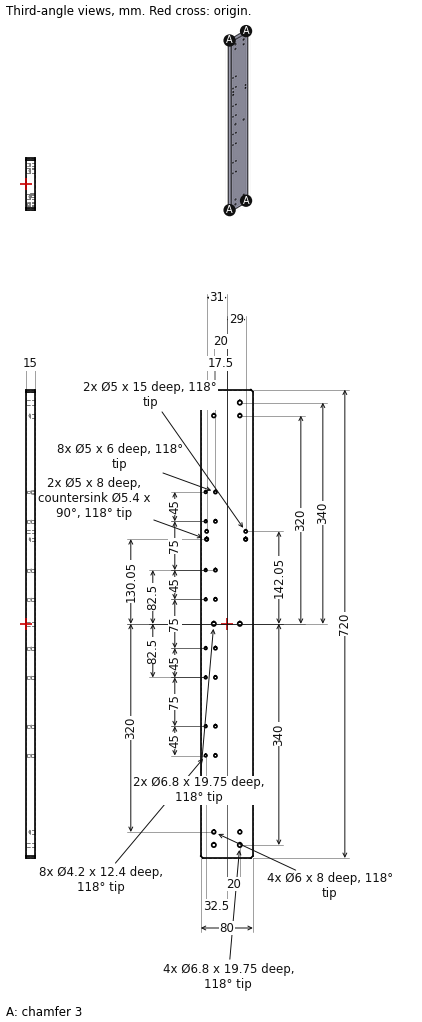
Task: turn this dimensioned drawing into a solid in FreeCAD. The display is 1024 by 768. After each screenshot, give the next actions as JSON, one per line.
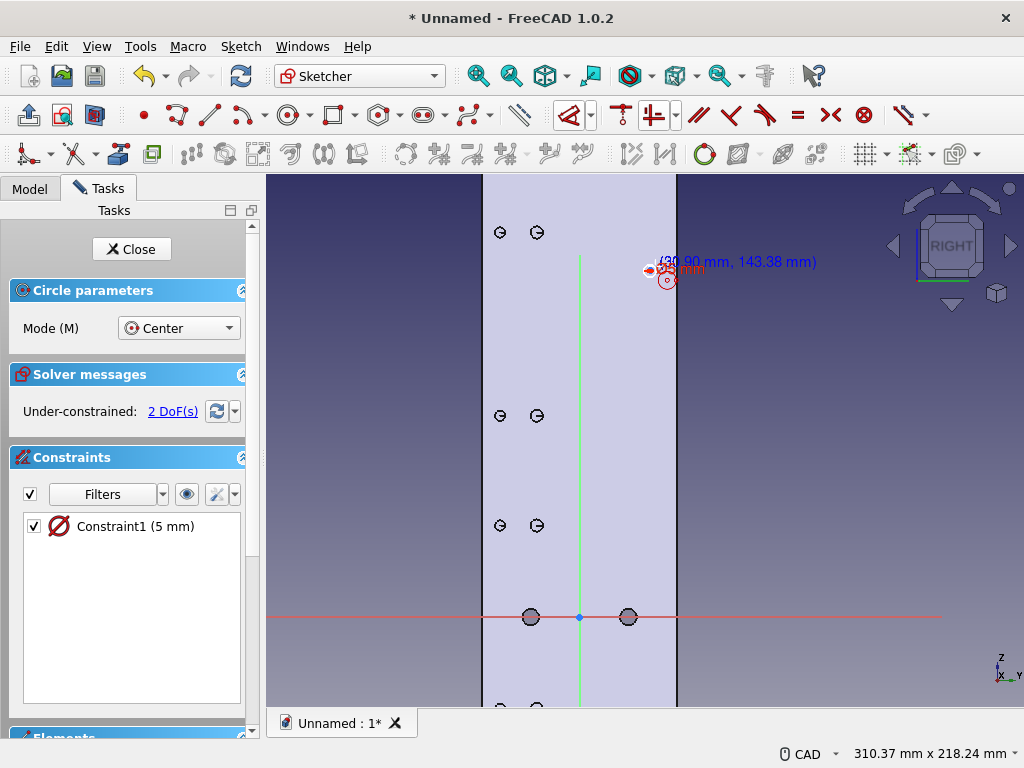
{"action": "scroll", "coordinate": [504, 270], "scroll_direction": "up", "scroll_amount": 7}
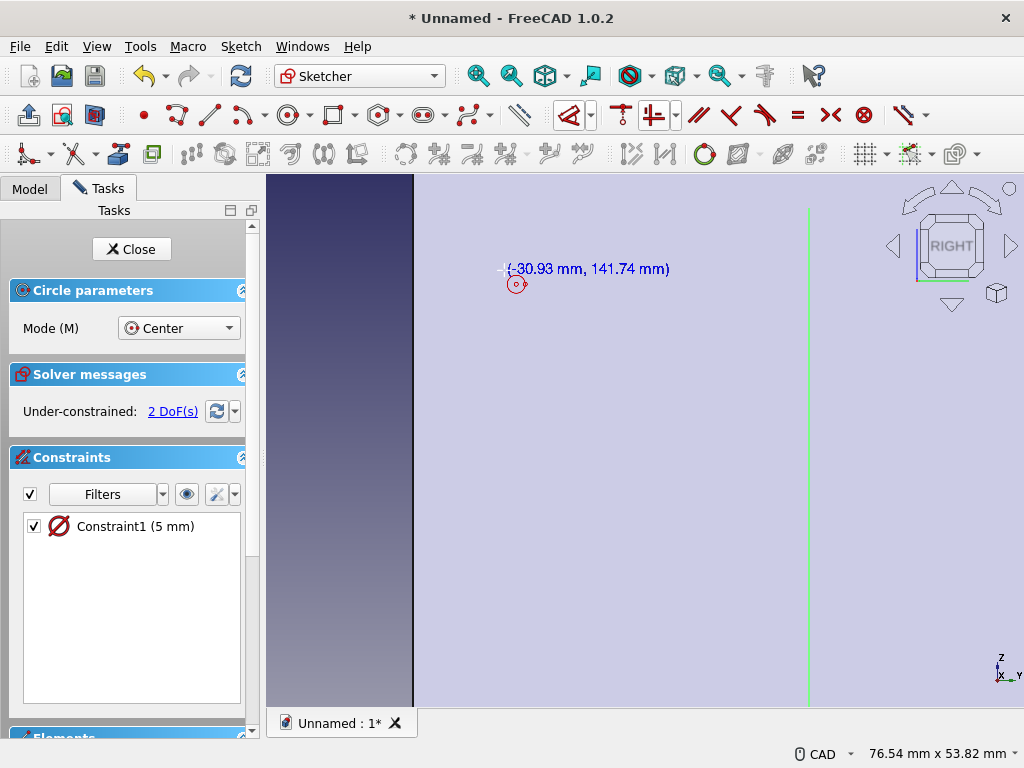
{"action": "scroll", "coordinate": [504, 270], "scroll_direction": "down", "scroll_amount": 7}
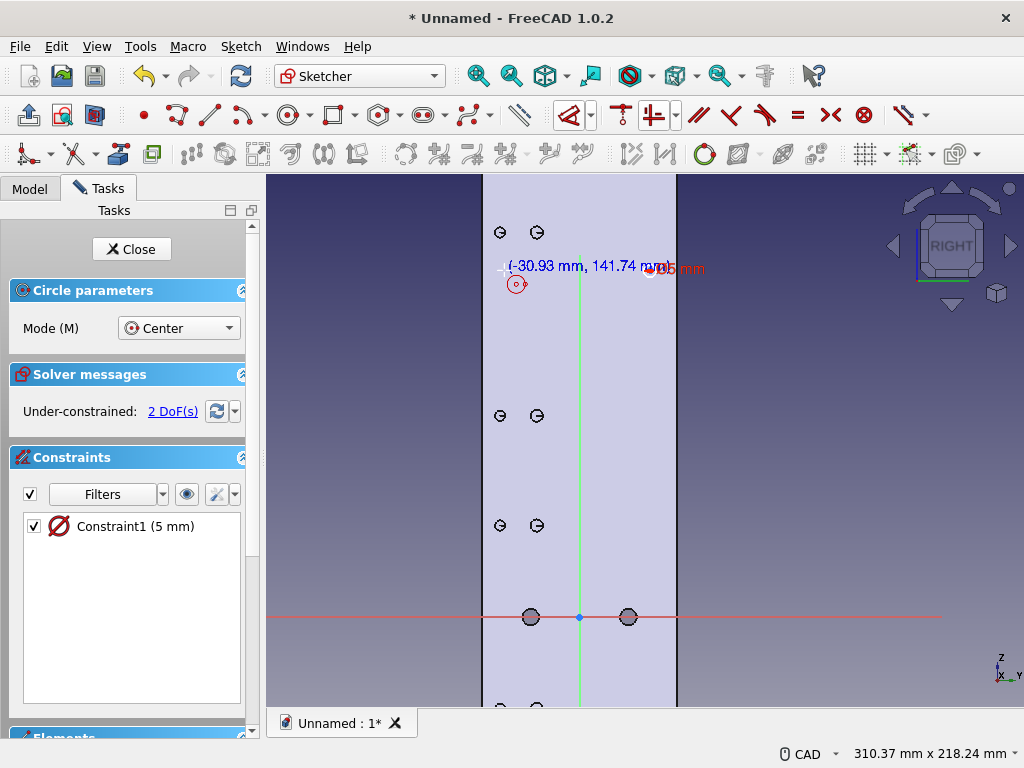
{"action": "left_click", "coordinate": [504, 270]}
{"action": "mouse_move", "coordinate": [508, 266]}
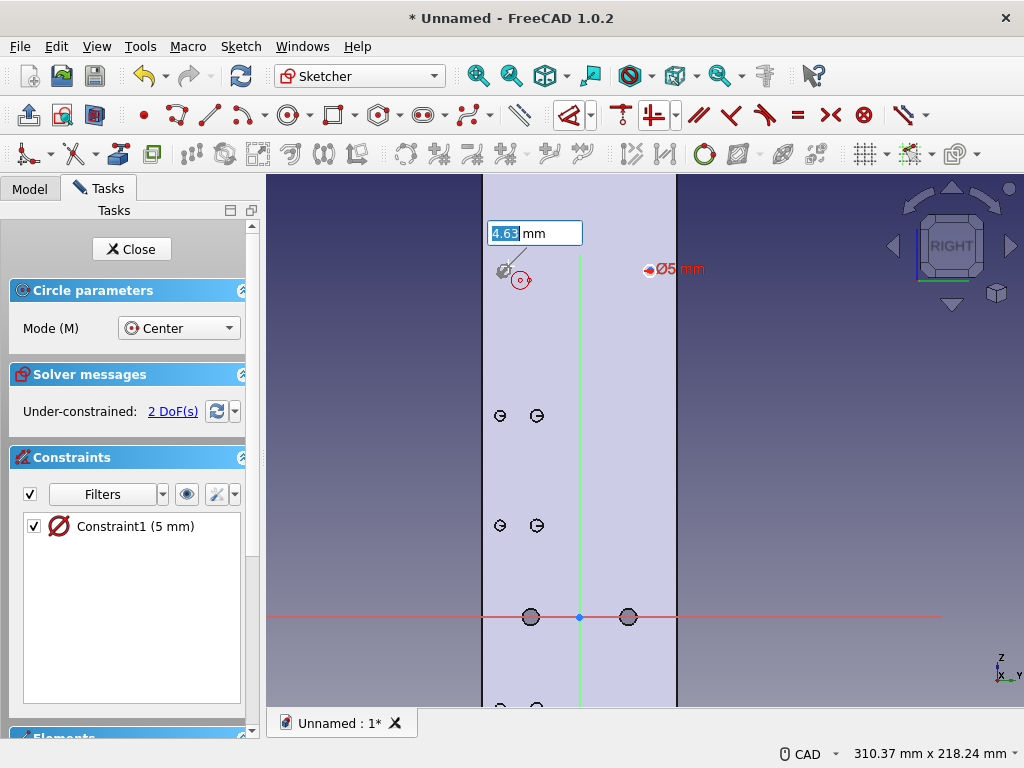
{"action": "type", "text": "5"}
{"action": "key", "text": "Return"}
{"action": "key", "text": "Escape"}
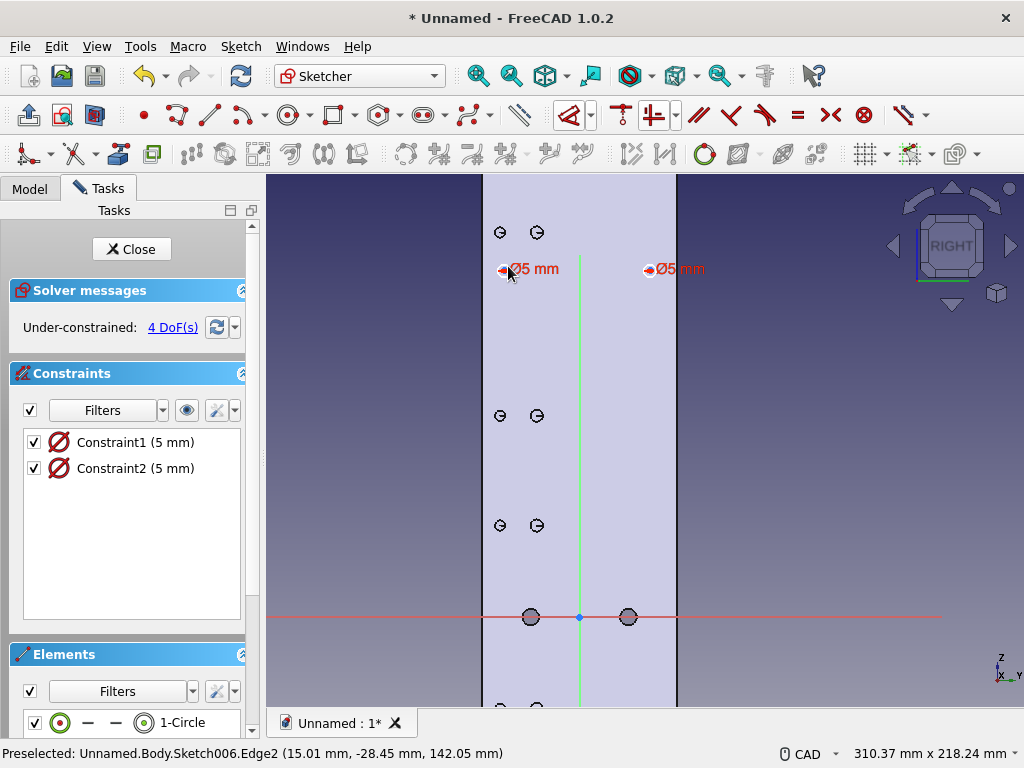
{"action": "left_click", "coordinate": [650, 271]}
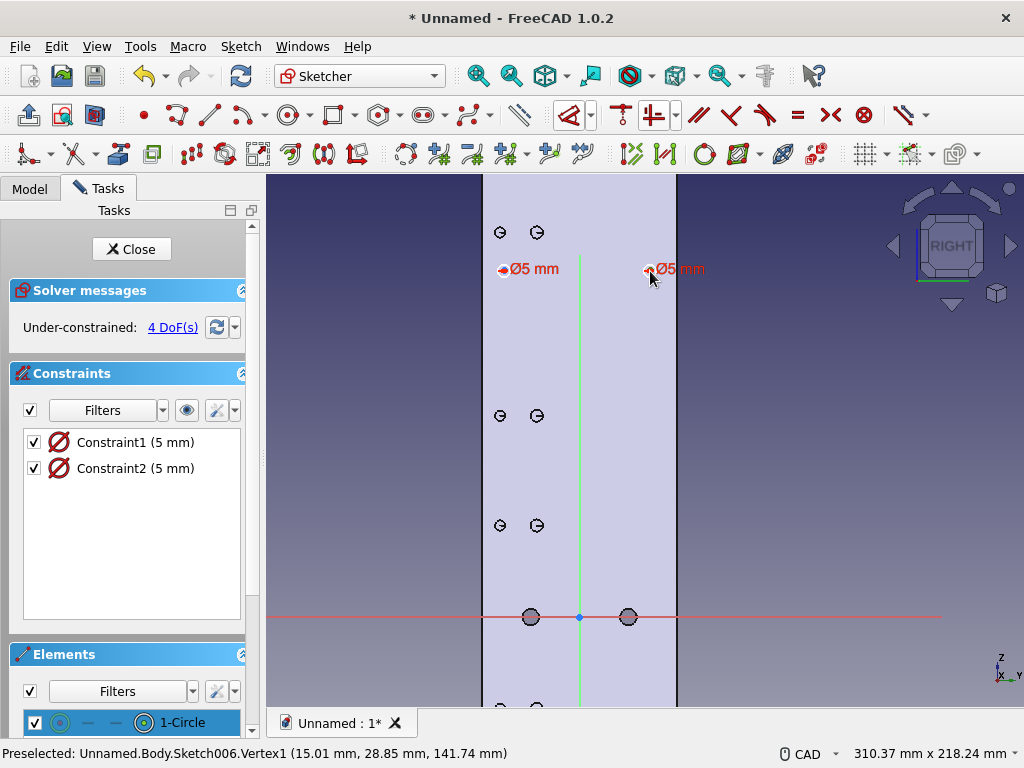
{"action": "left_click", "coordinate": [504, 271]}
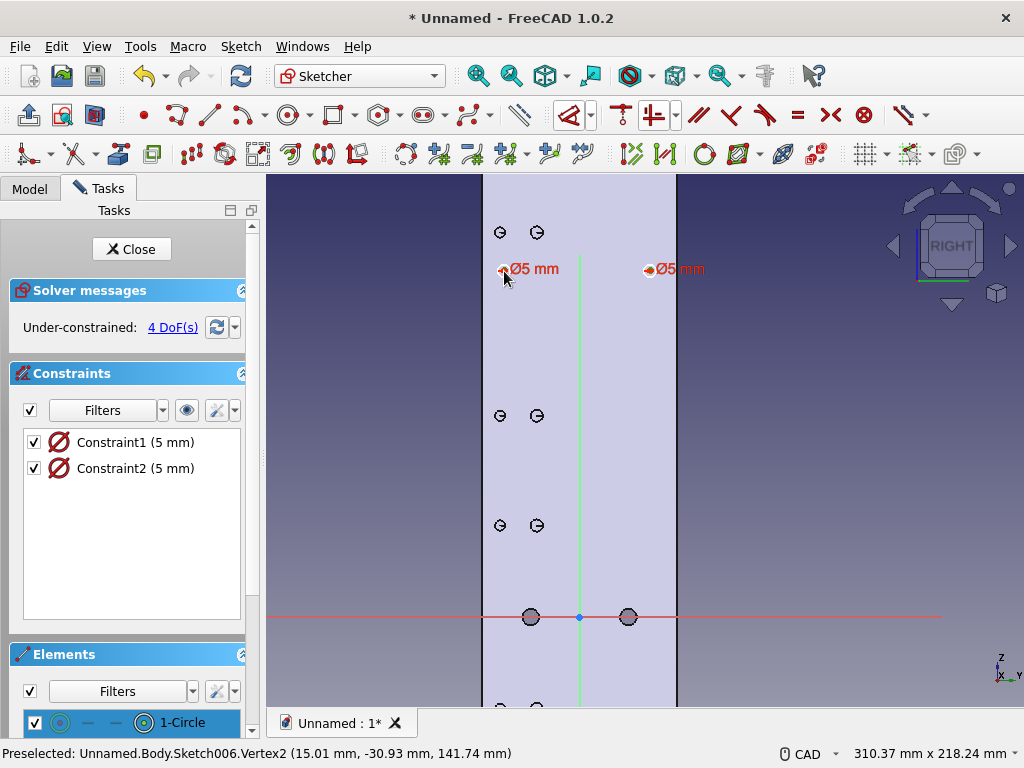
{"action": "key", "text": "h"}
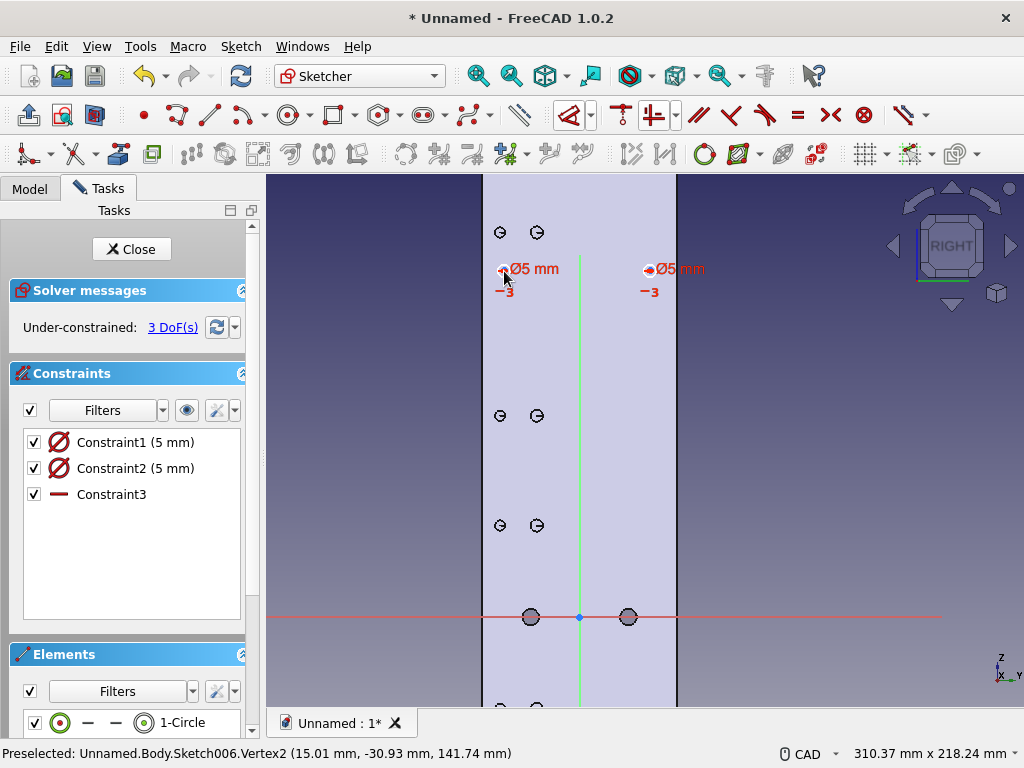
{"action": "left_click", "coordinate": [650, 271]}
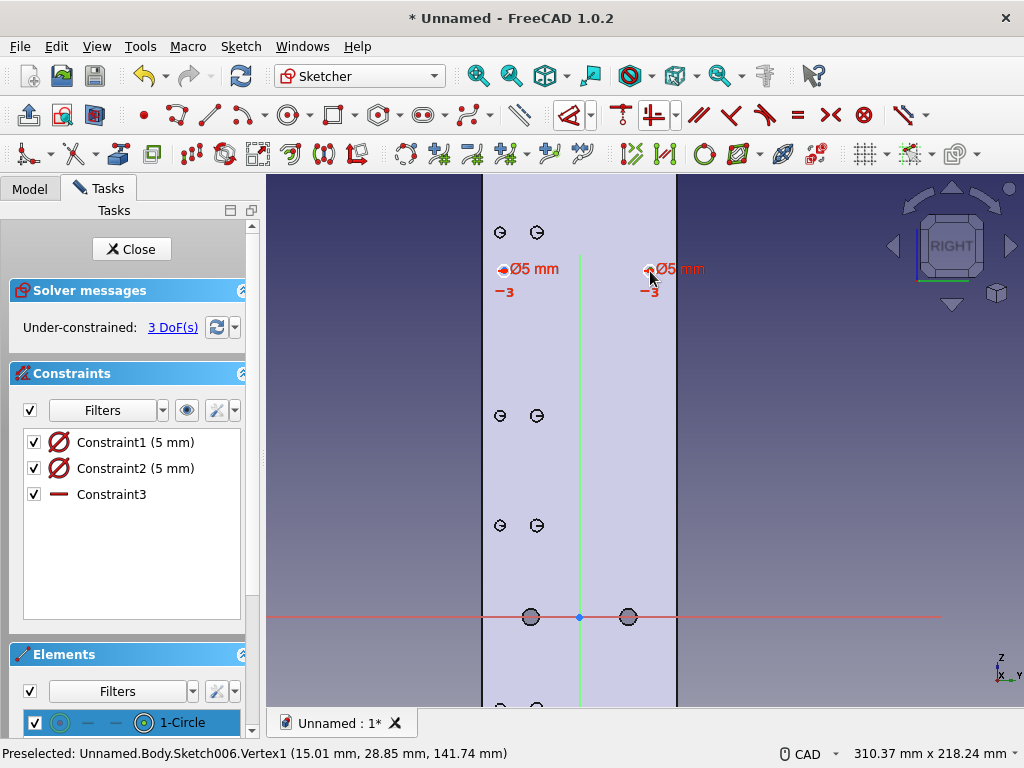
{"action": "key", "text": "l"}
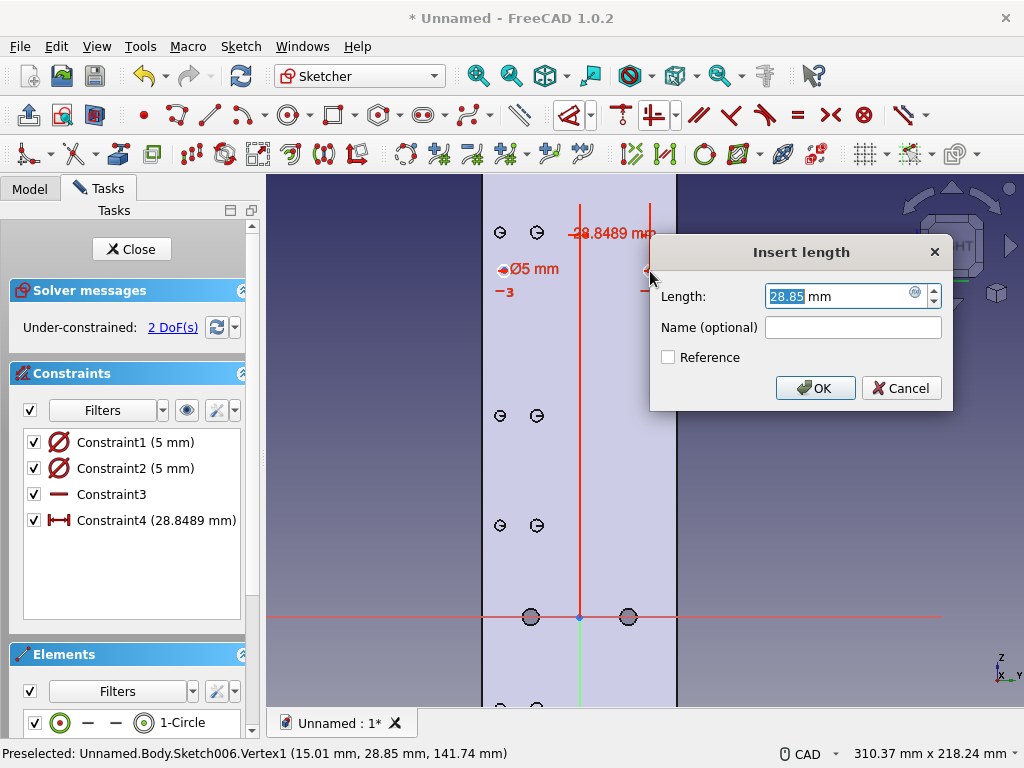
{"action": "type", "text": "29"}
{"action": "key", "text": "Return"}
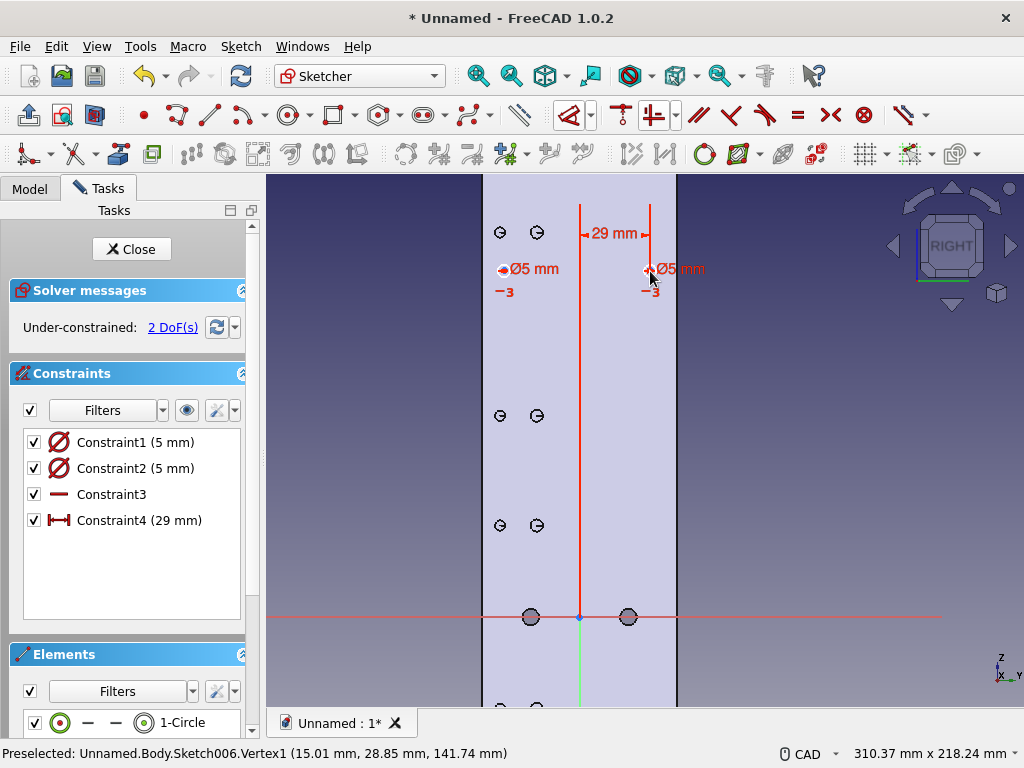
{"action": "left_click", "coordinate": [504, 271]}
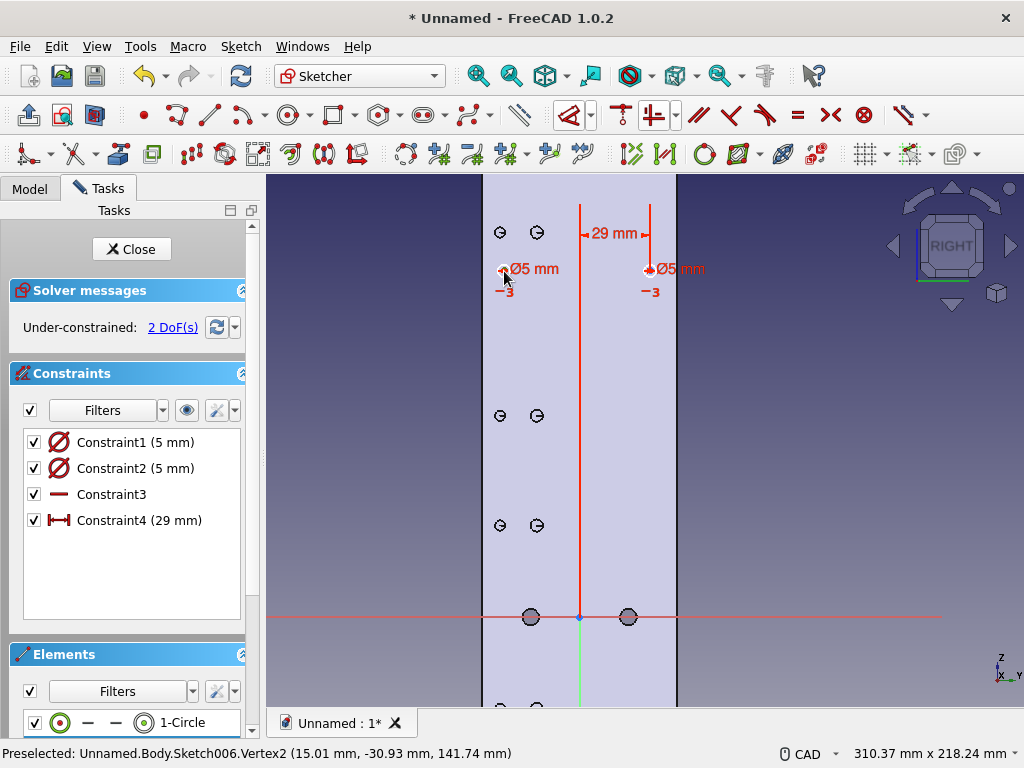
{"action": "left_click", "coordinate": [590, 116]}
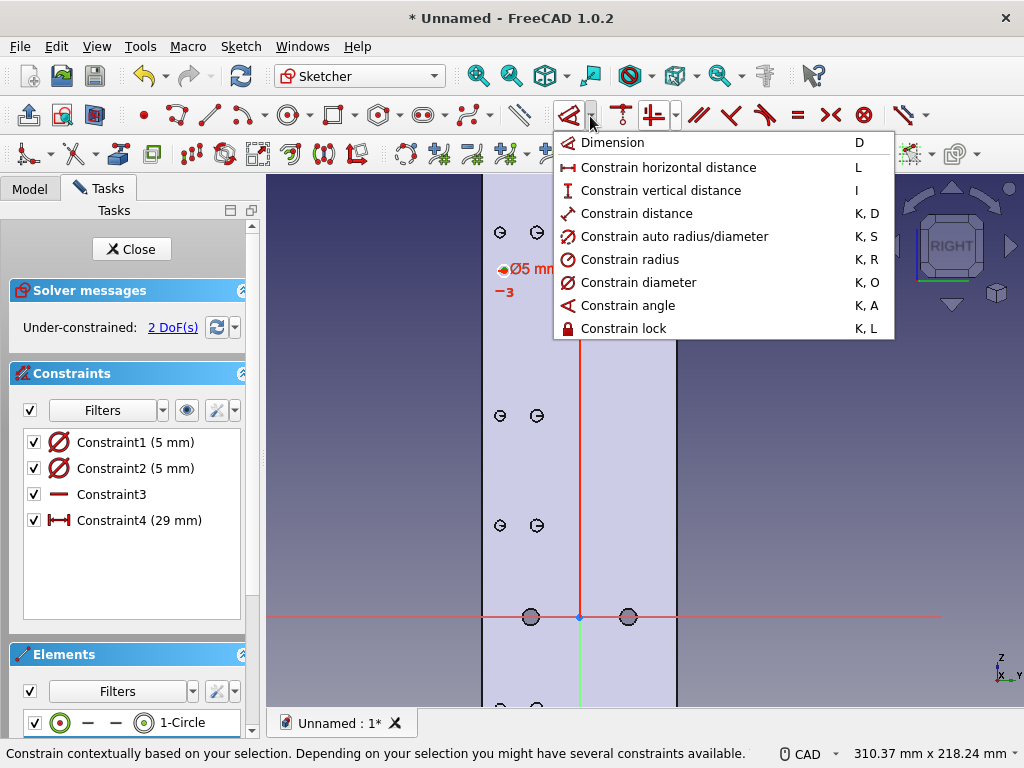
{"action": "left_click", "coordinate": [724, 168]}